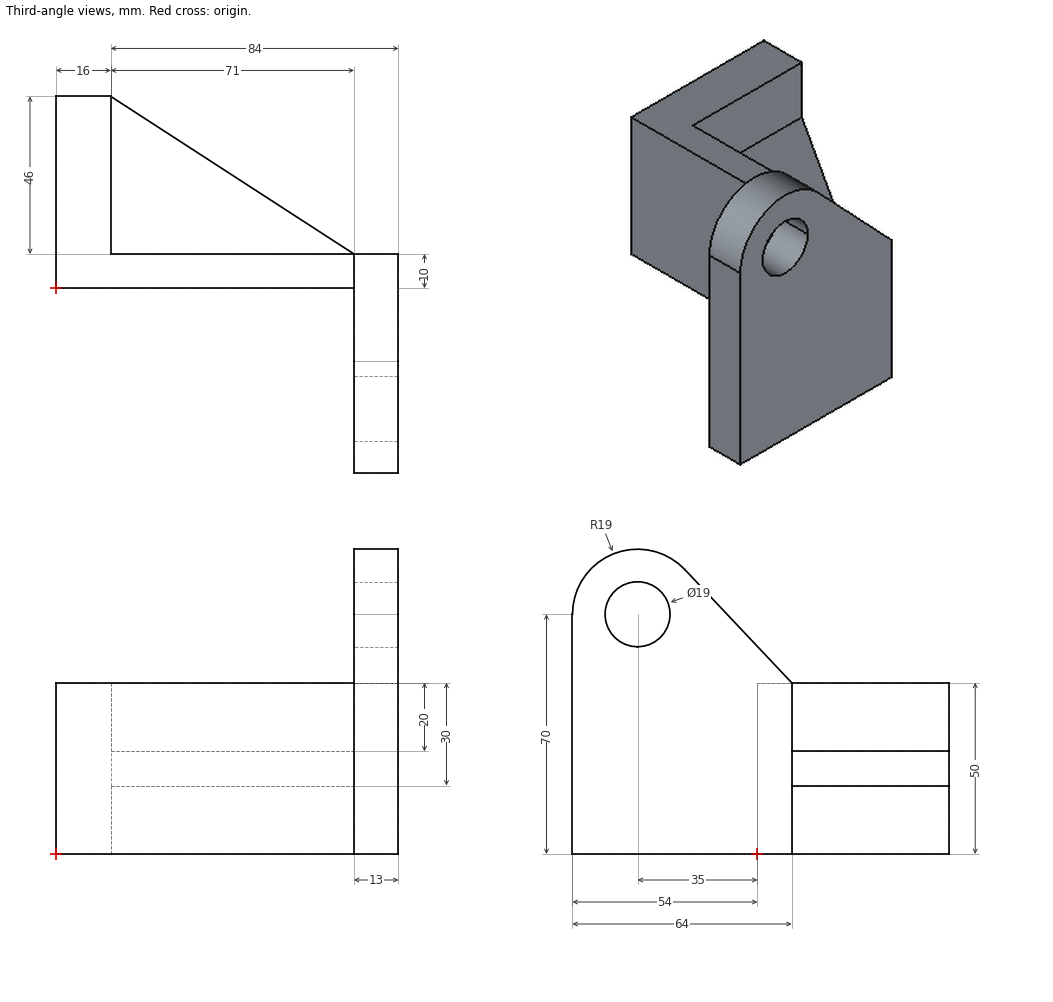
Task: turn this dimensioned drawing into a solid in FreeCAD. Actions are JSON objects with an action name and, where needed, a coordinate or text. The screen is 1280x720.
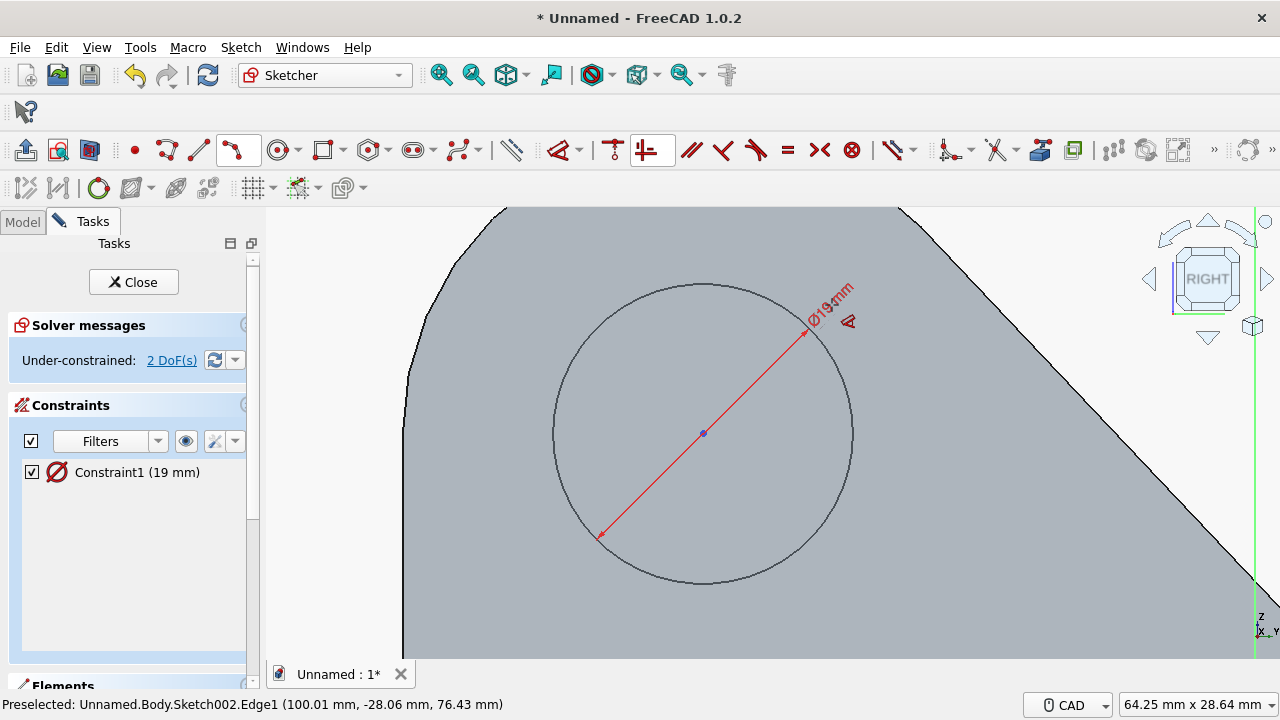
{"action": "left_click", "coordinate": [703, 434]}
{"action": "left_click", "coordinate": [909, 400]}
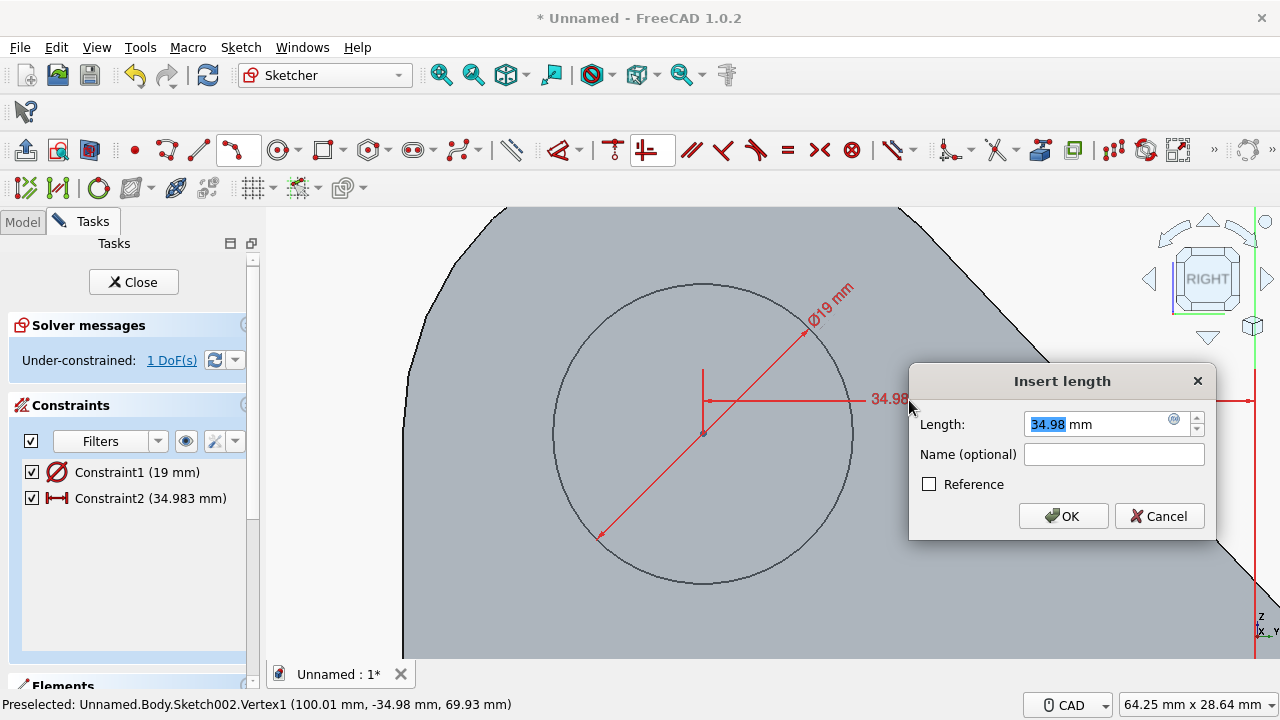
{"action": "type", "text": "35"}
{"action": "key", "text": "Return"}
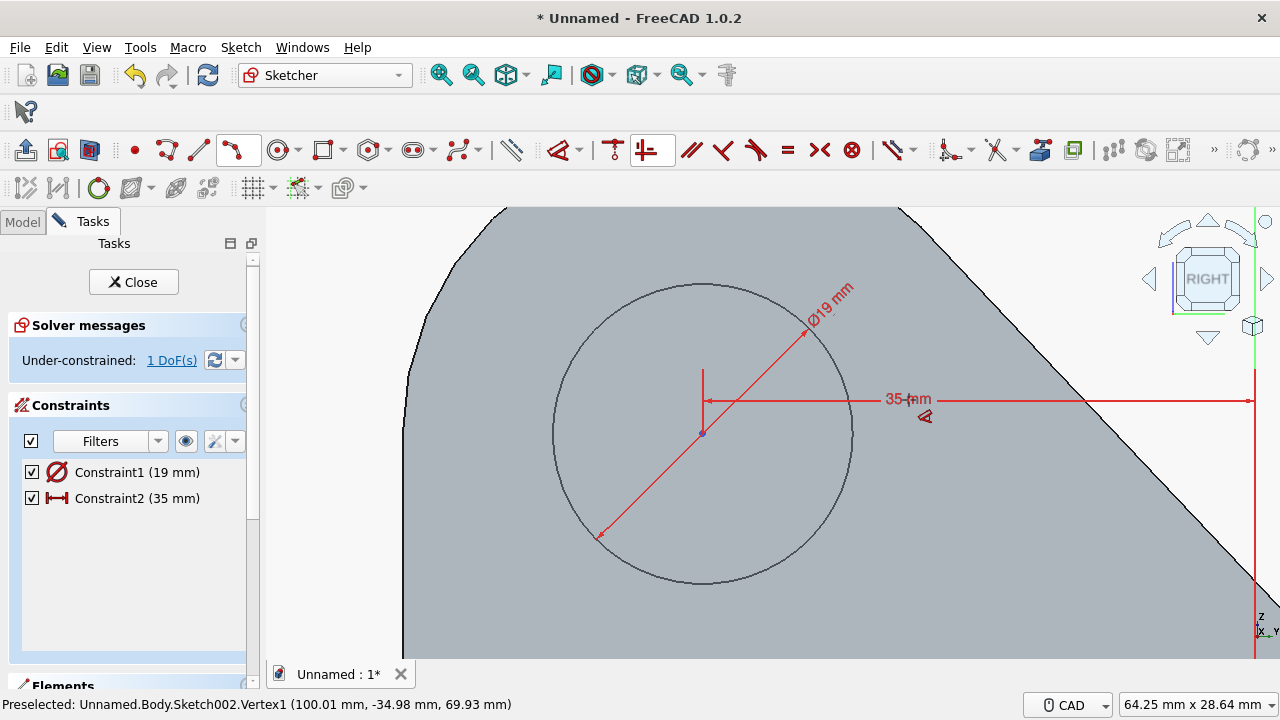
{"action": "left_click", "coordinate": [703, 434]}
{"action": "left_click", "coordinate": [669, 532]}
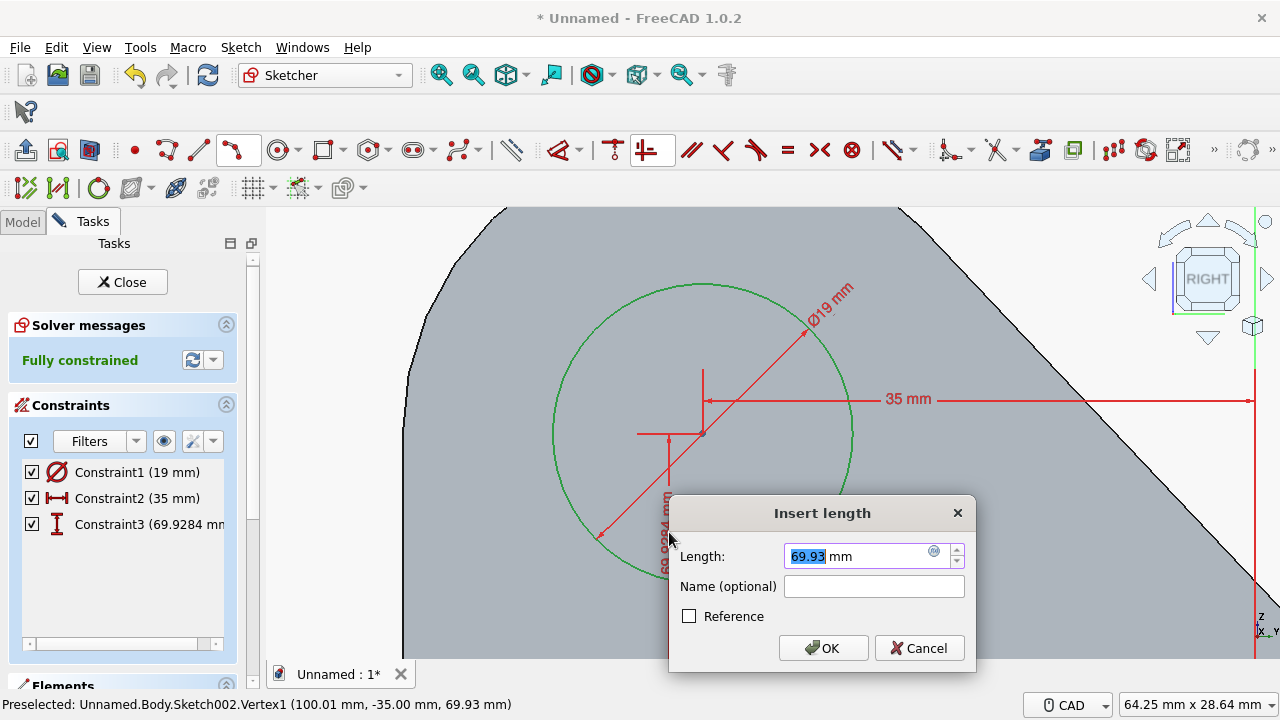
{"action": "type", "text": "70"}
{"action": "key", "text": "Return"}
{"action": "key", "text": "Escape"}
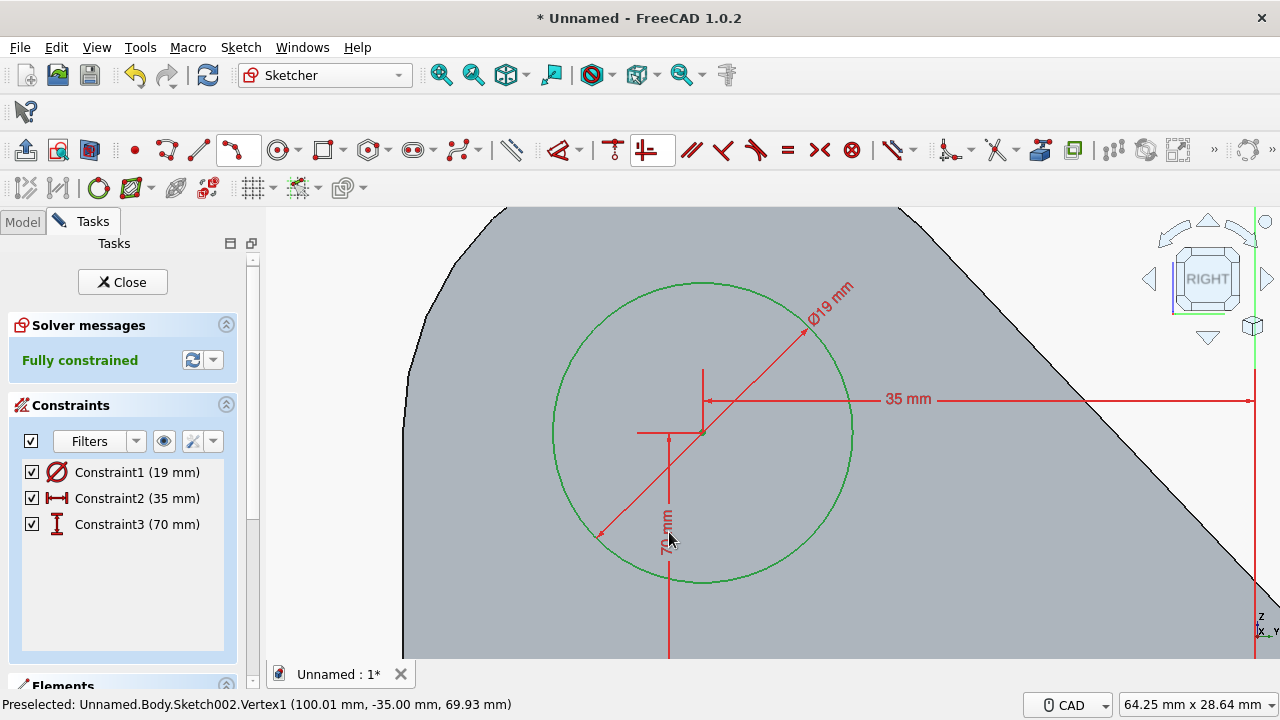
{"action": "left_click", "coordinate": [123, 282]}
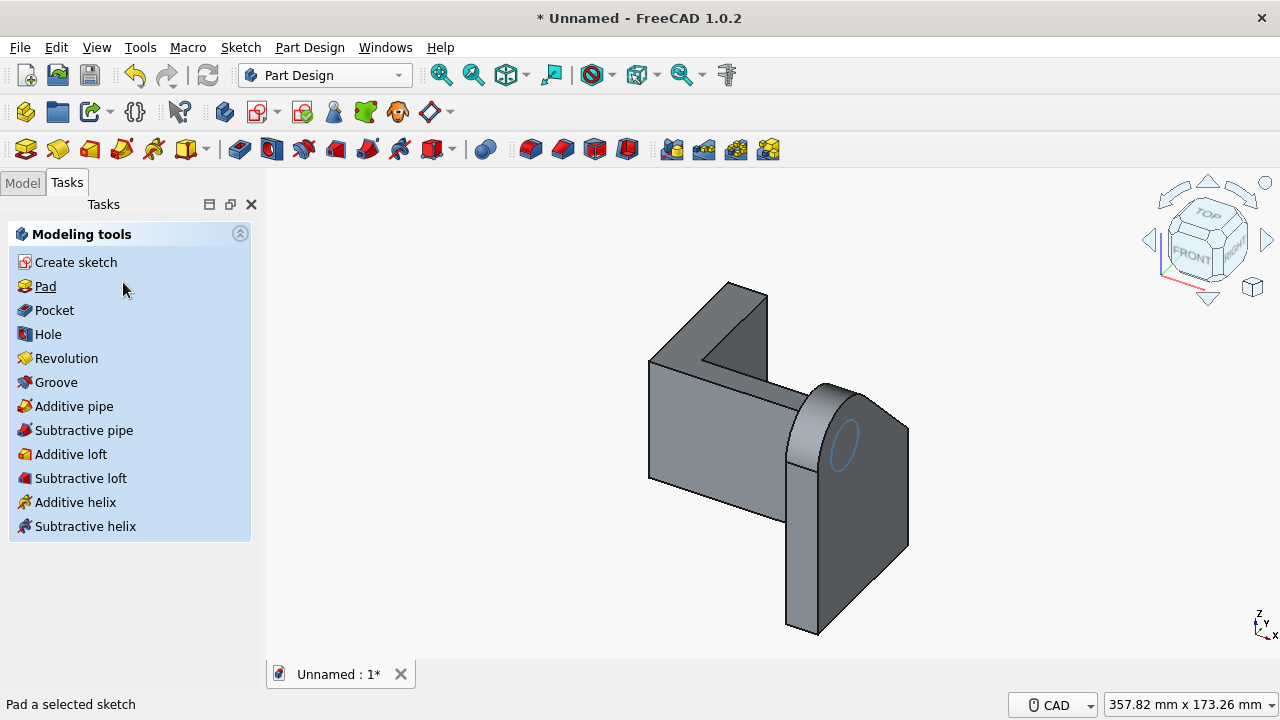
{"action": "left_click", "coordinate": [240, 150]}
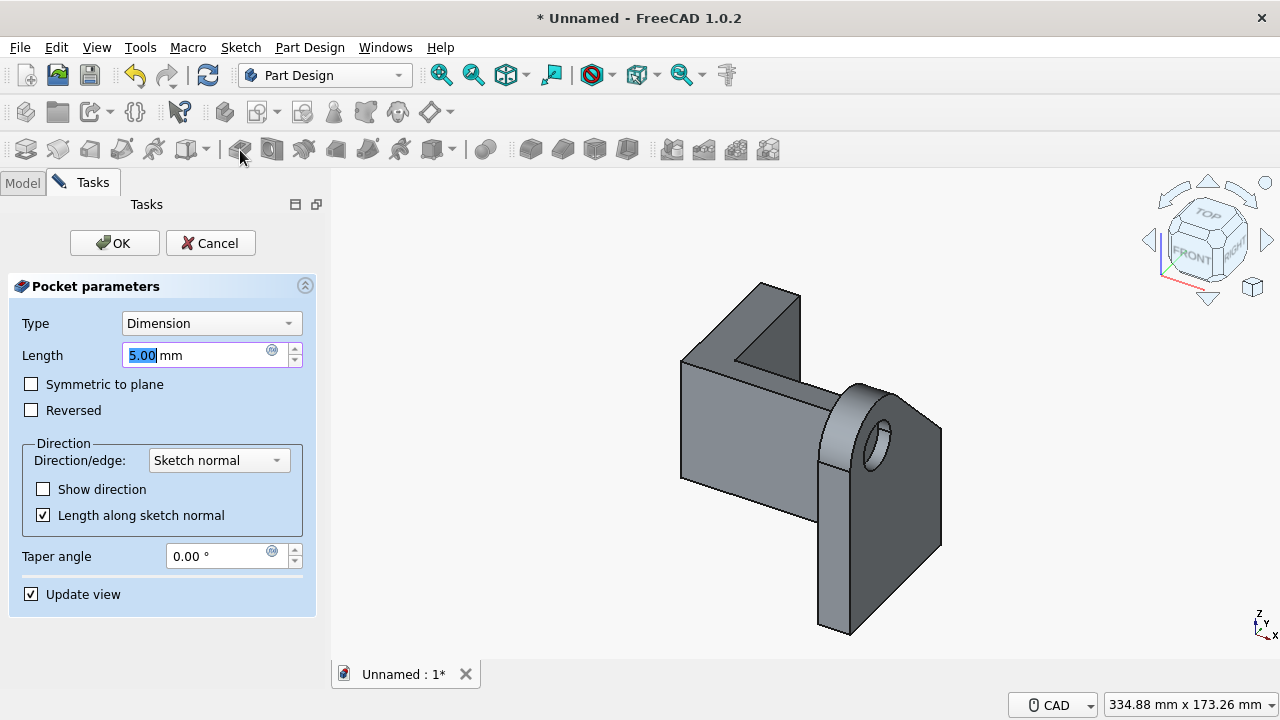
{"action": "type", "text": "13"}
{"action": "key", "text": "Tab"}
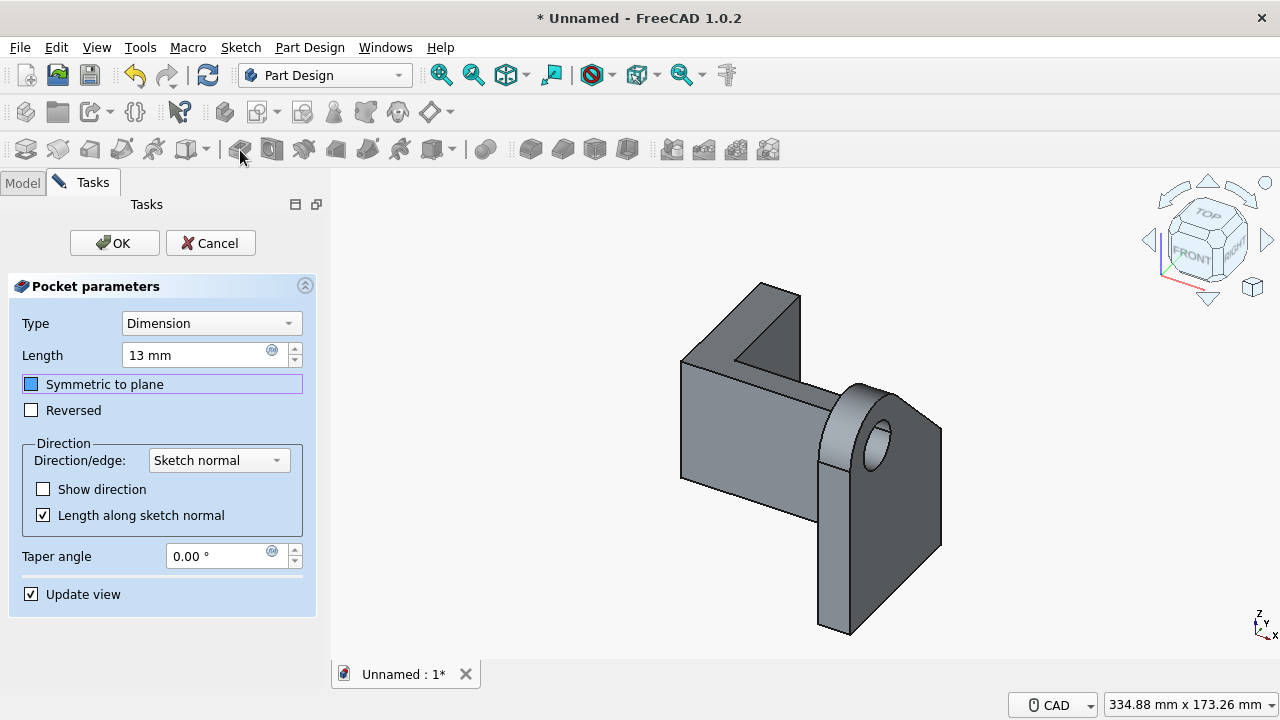
{"action": "left_click", "coordinate": [115, 243]}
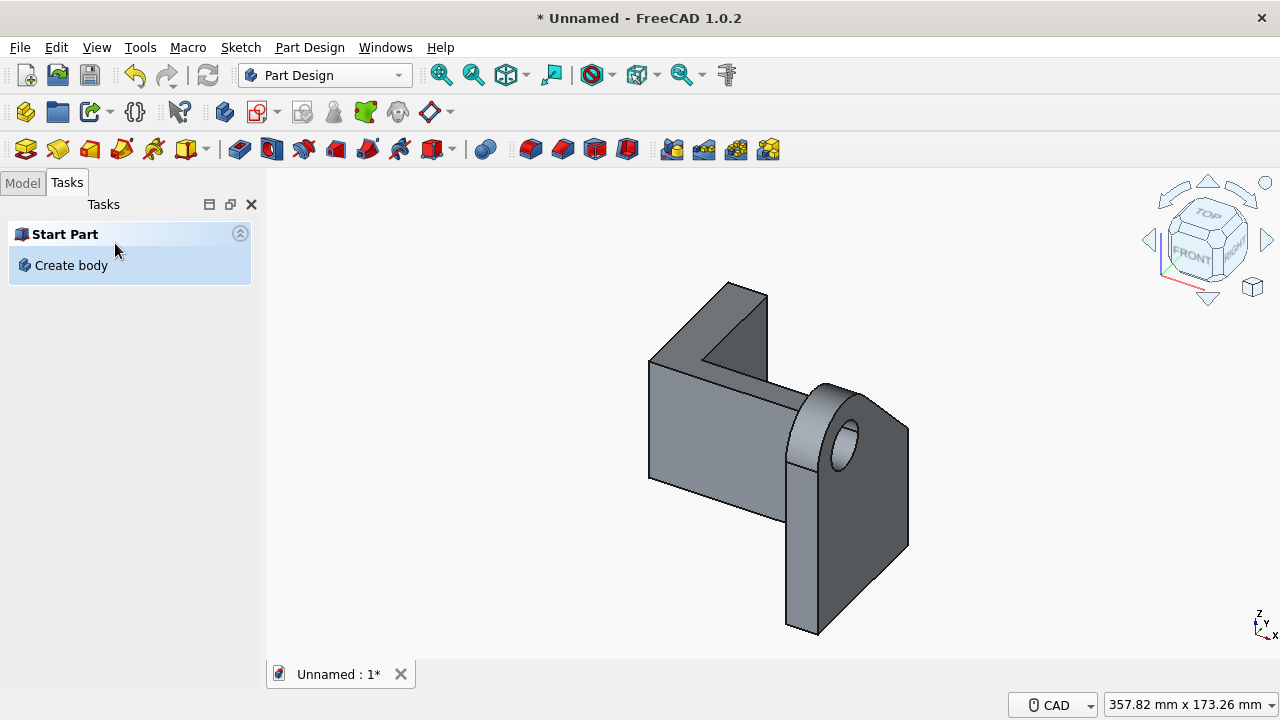
{"action": "left_click", "coordinate": [726, 304]}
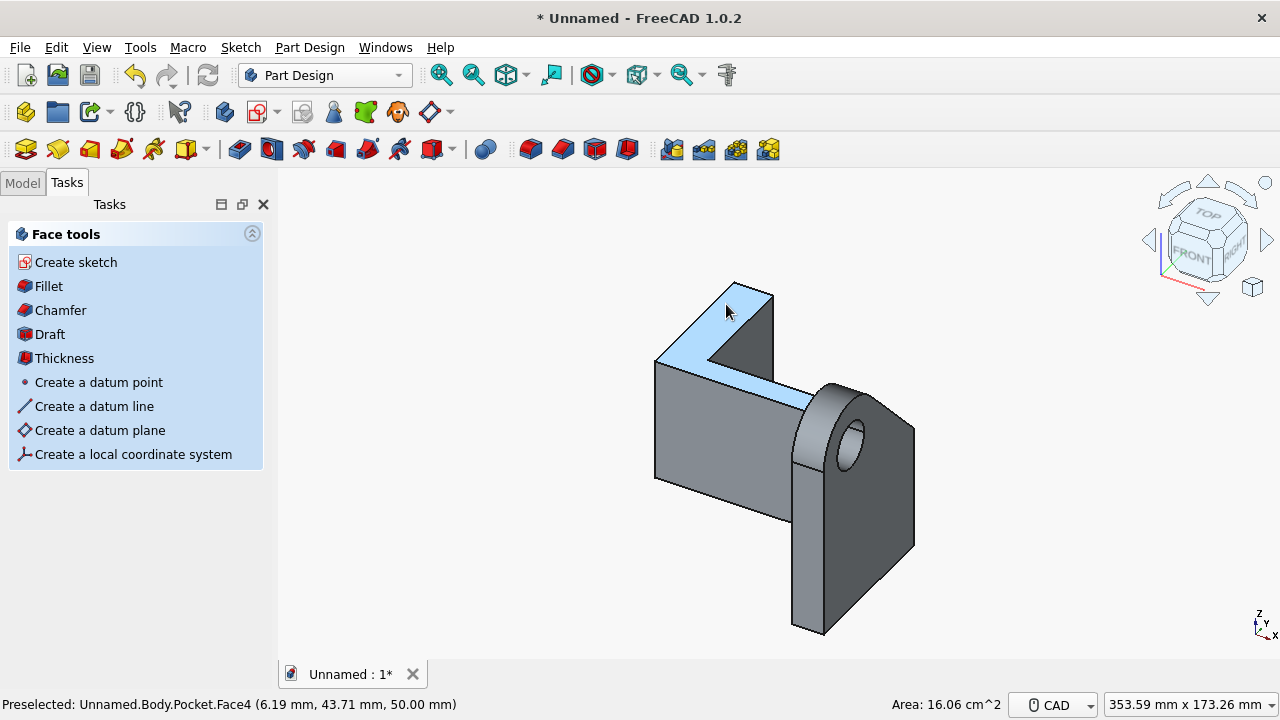
{"action": "left_click", "coordinate": [258, 112]}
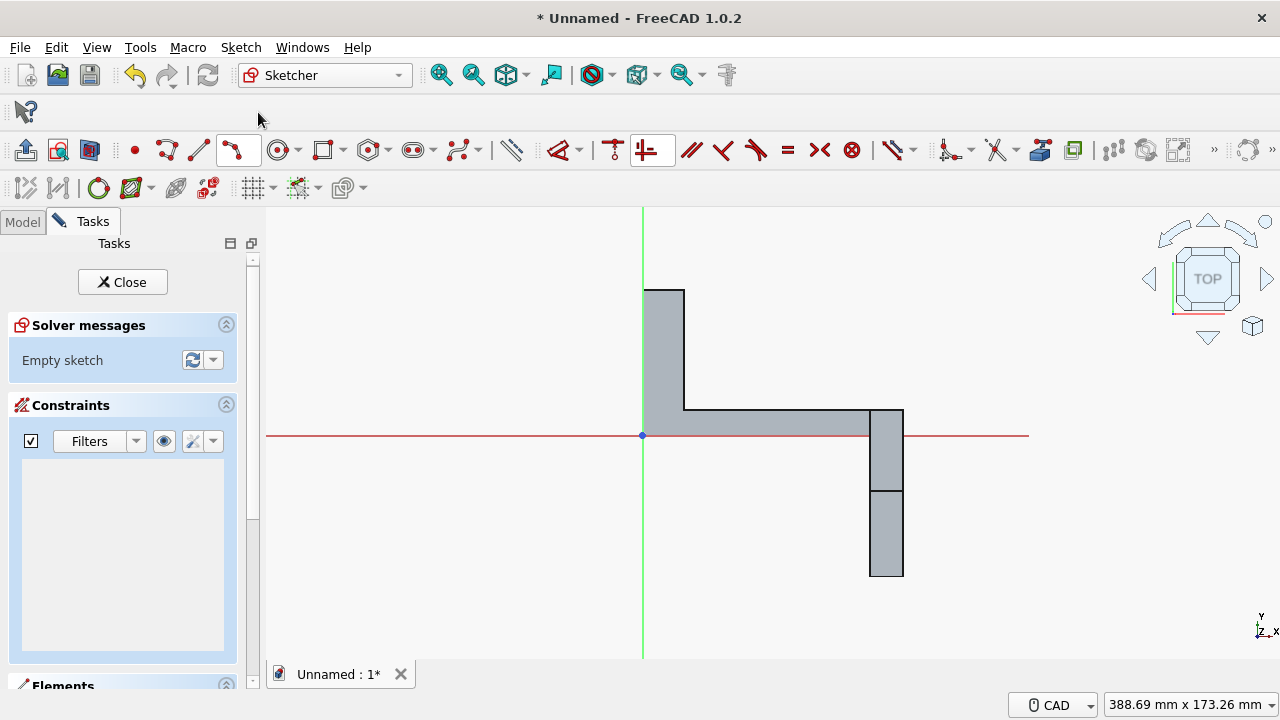
{"action": "left_click", "coordinate": [90, 150]}